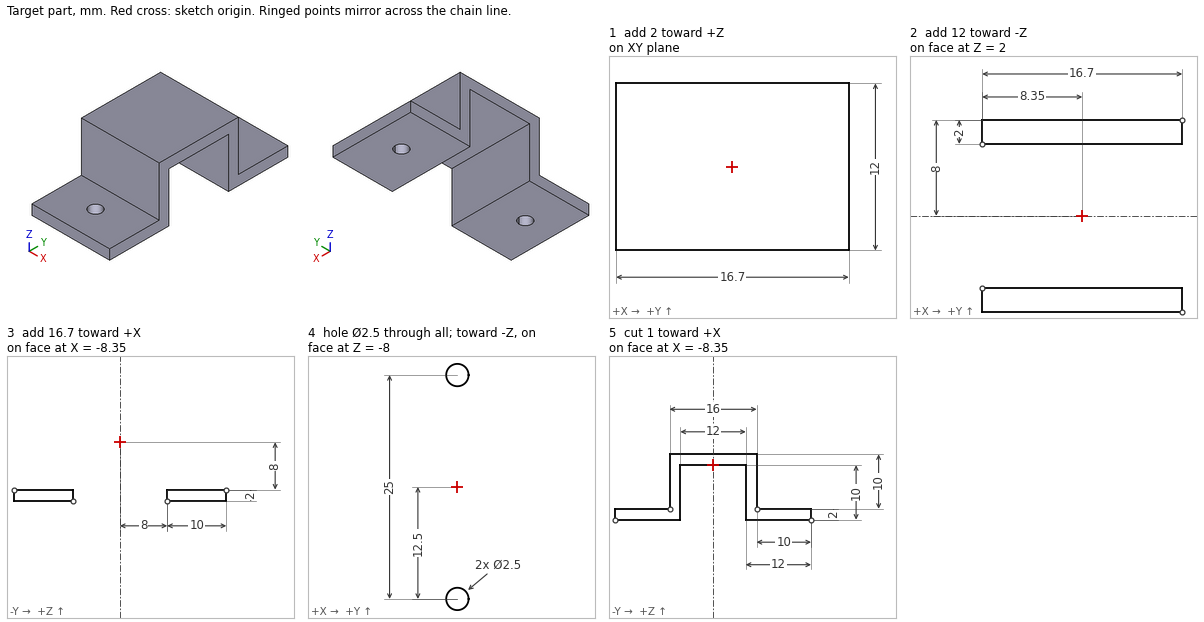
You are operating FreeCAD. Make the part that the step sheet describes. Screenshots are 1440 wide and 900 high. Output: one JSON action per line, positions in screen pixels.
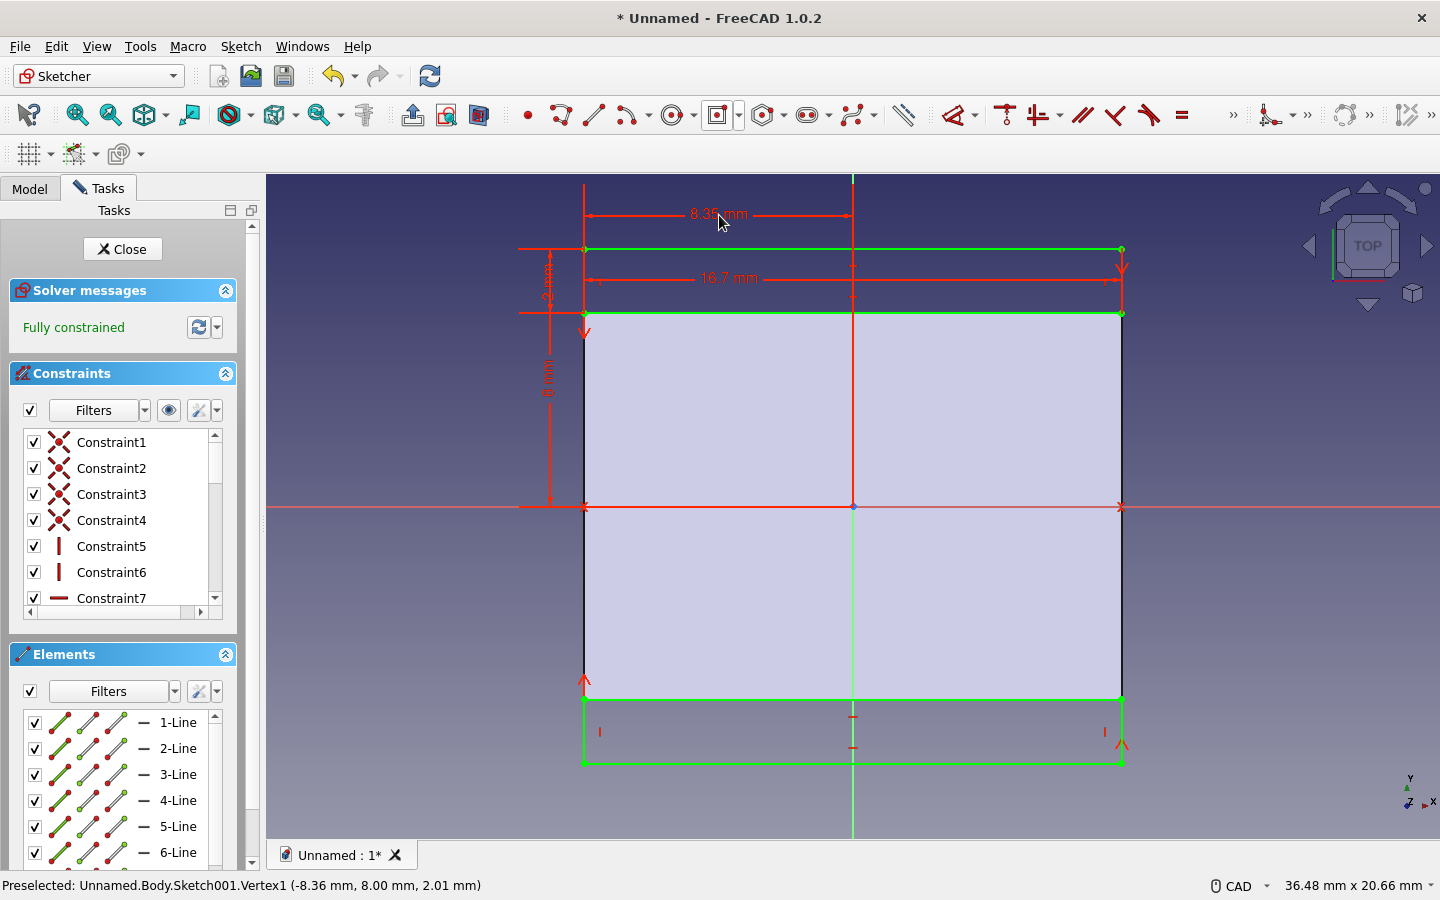
{"action": "left_click", "coordinate": [123, 249]}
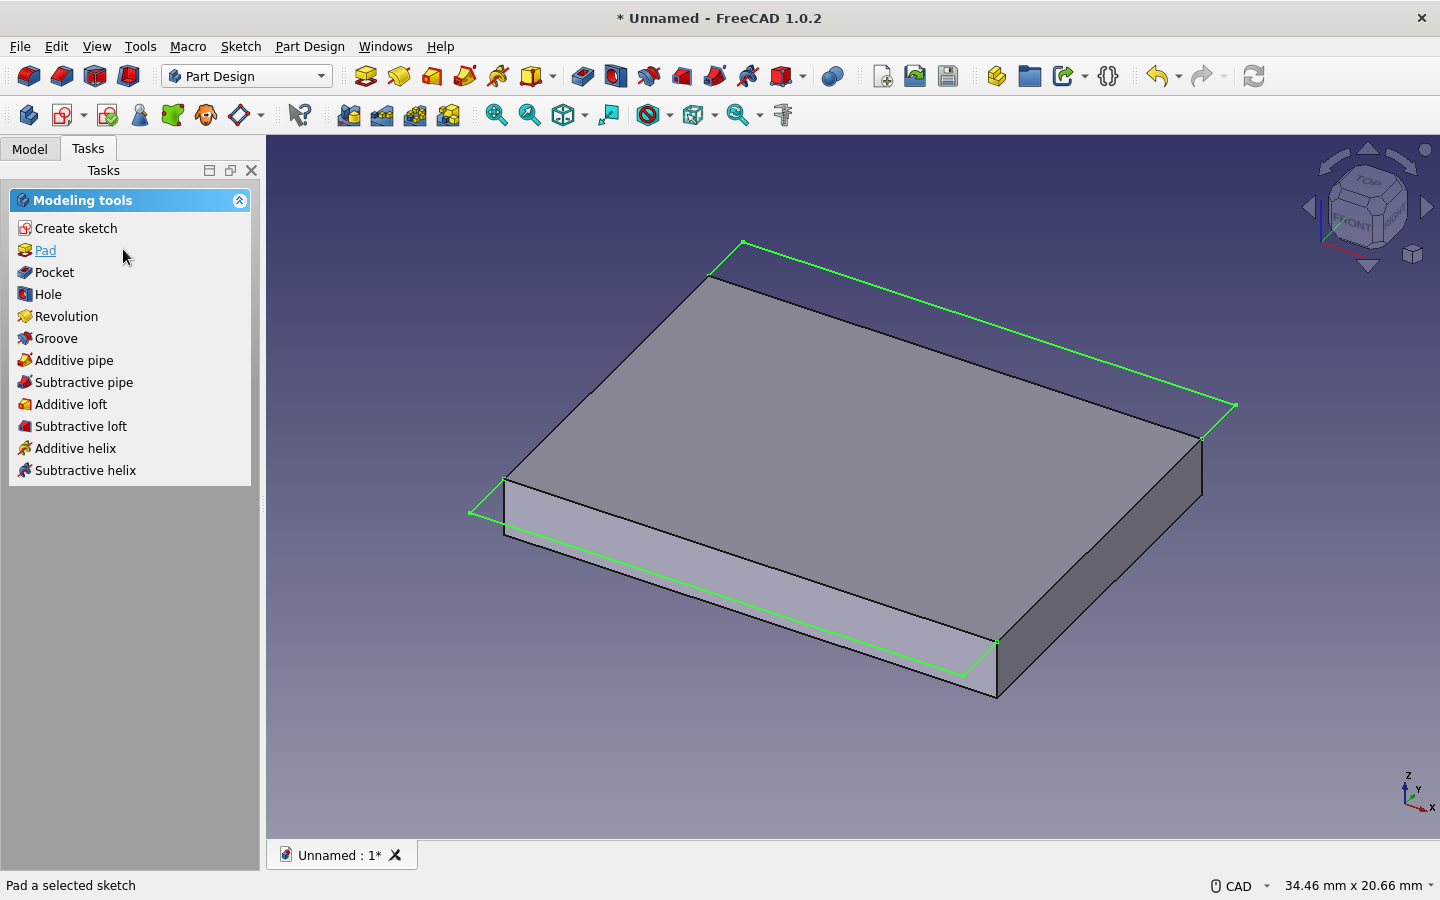
{"action": "left_click", "coordinate": [366, 76]}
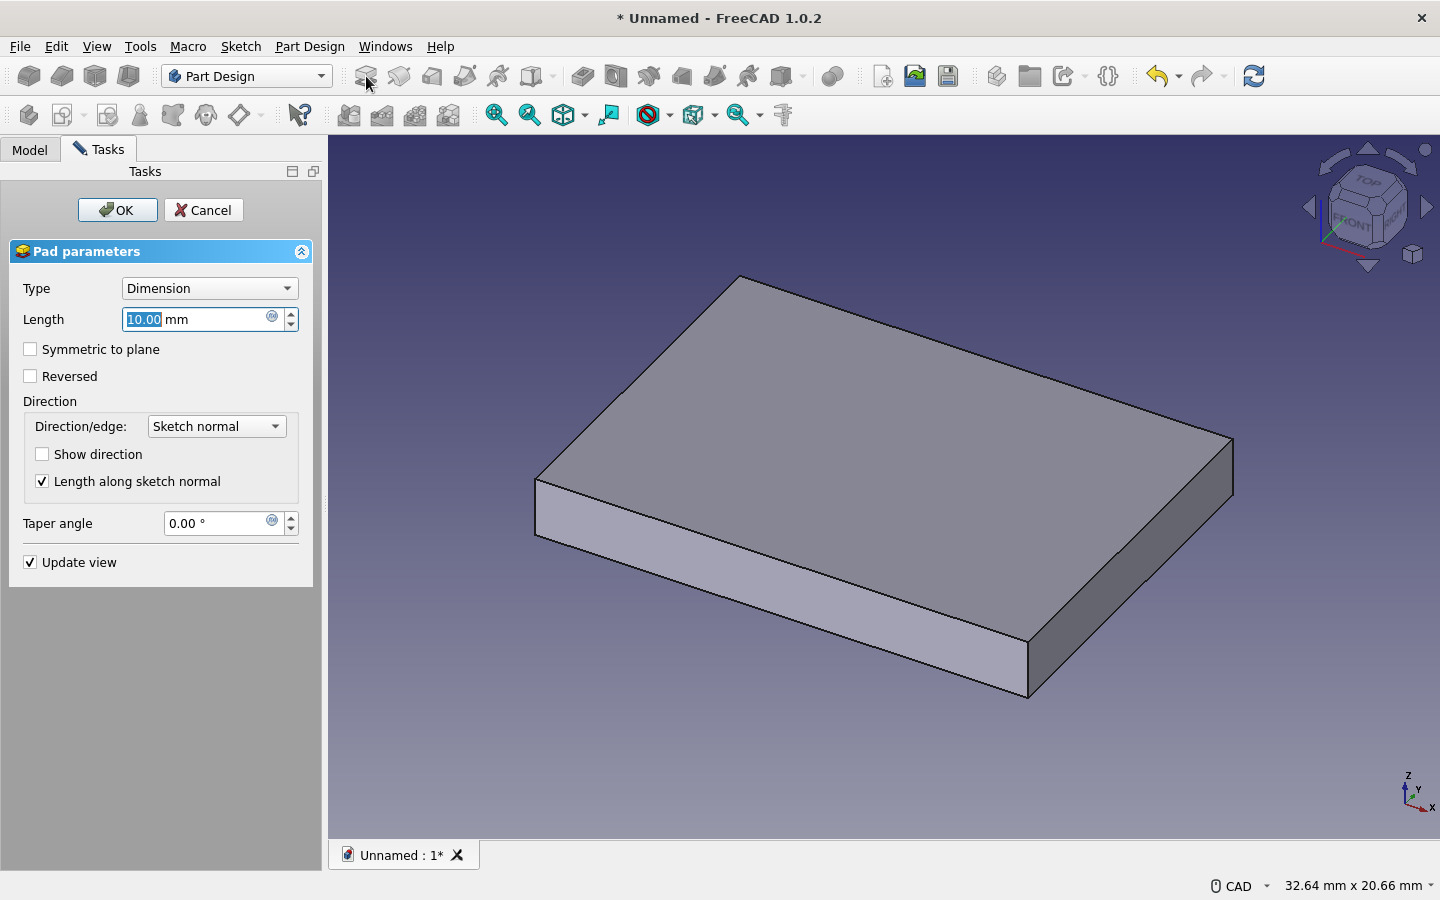
{"action": "type", "text": "12"}
{"action": "key", "text": "Tab"}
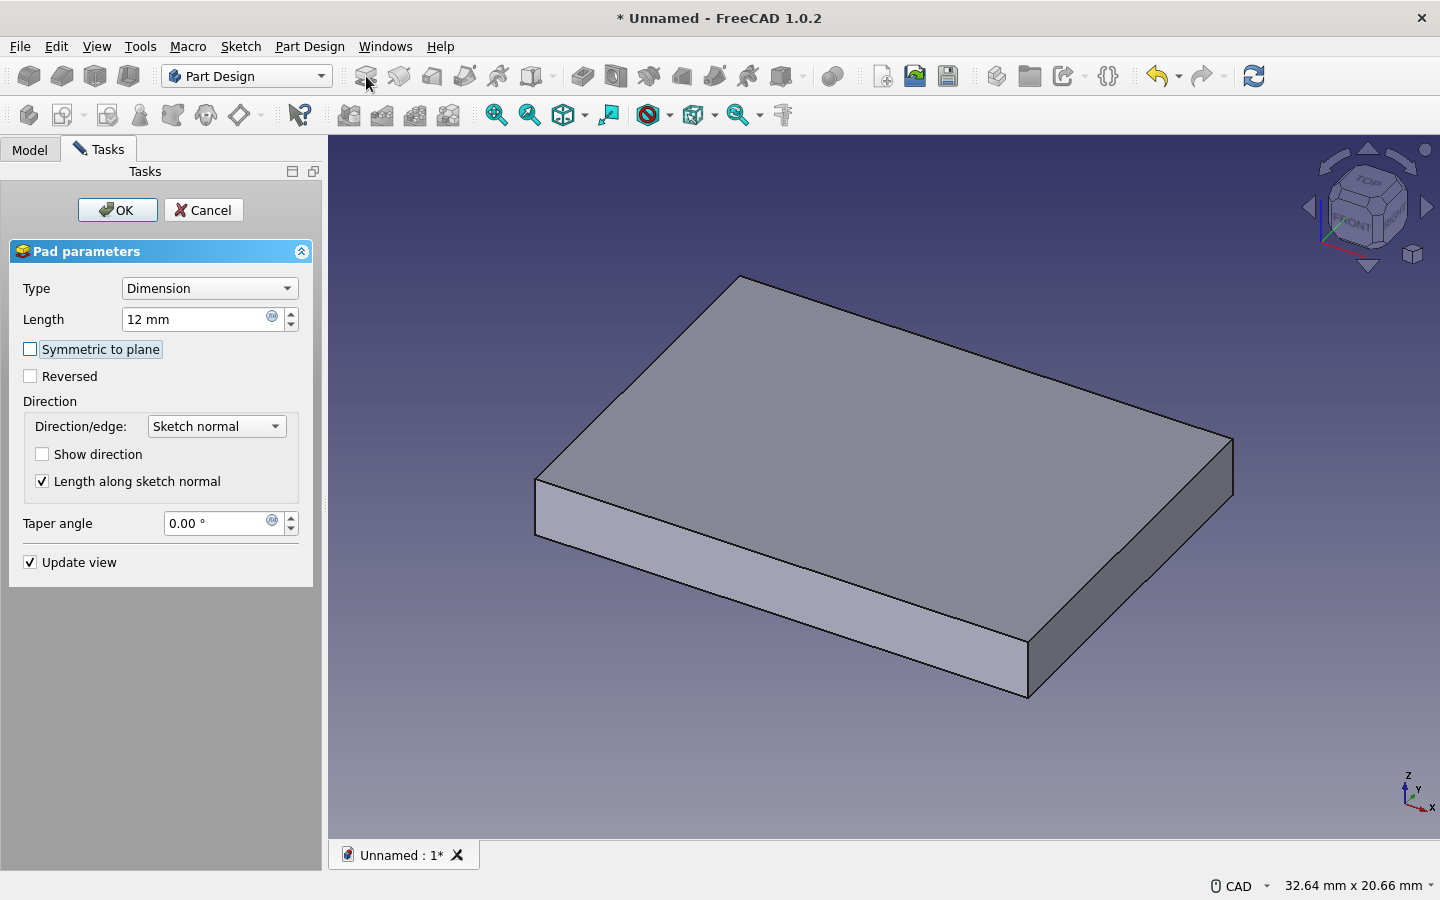
{"action": "left_click", "coordinate": [31, 376]}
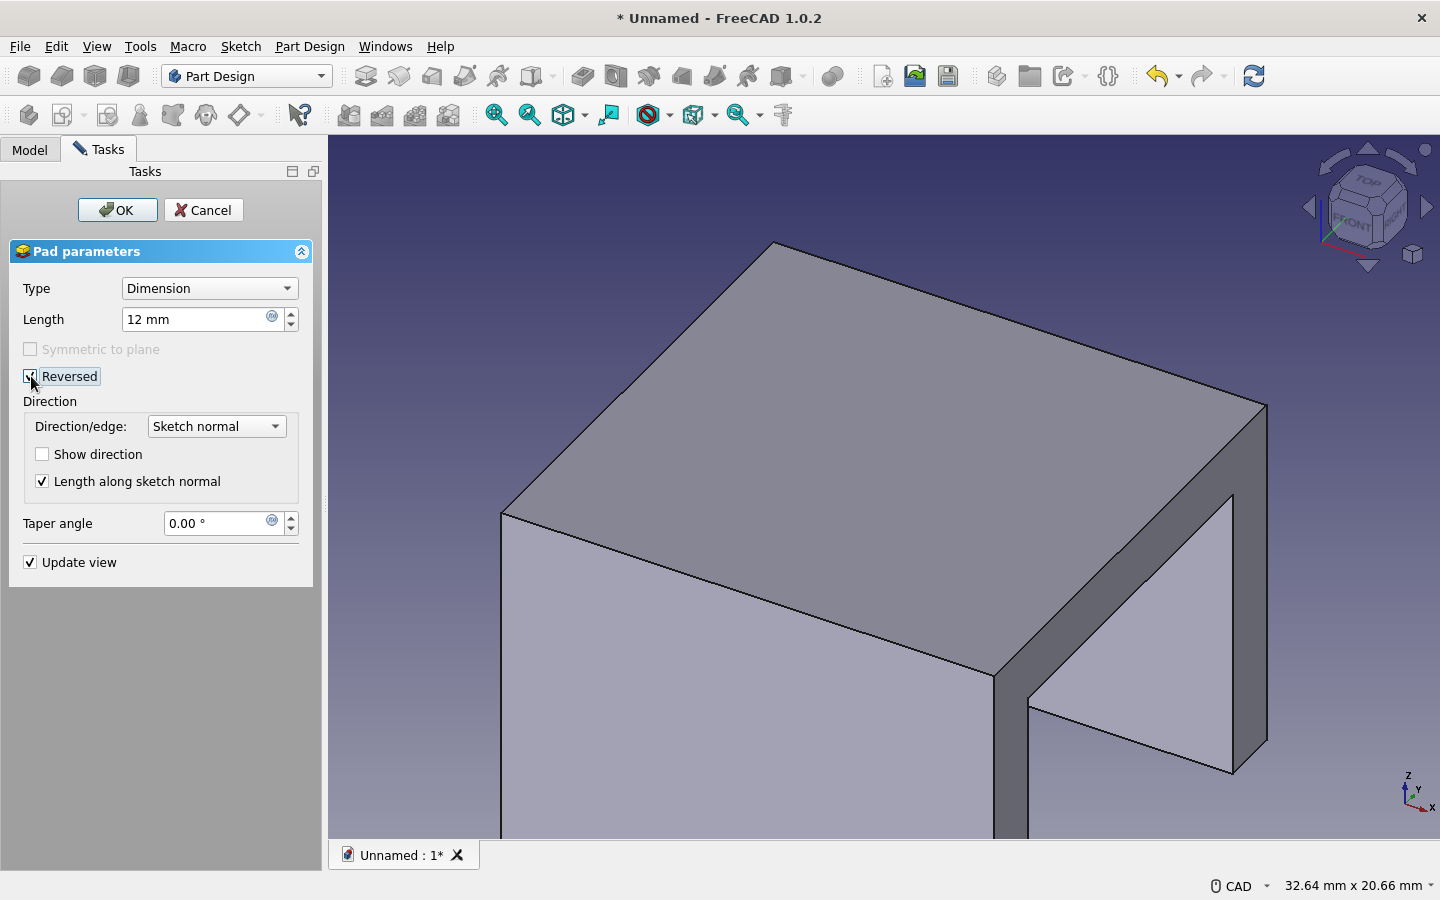
{"action": "left_click", "coordinate": [118, 210]}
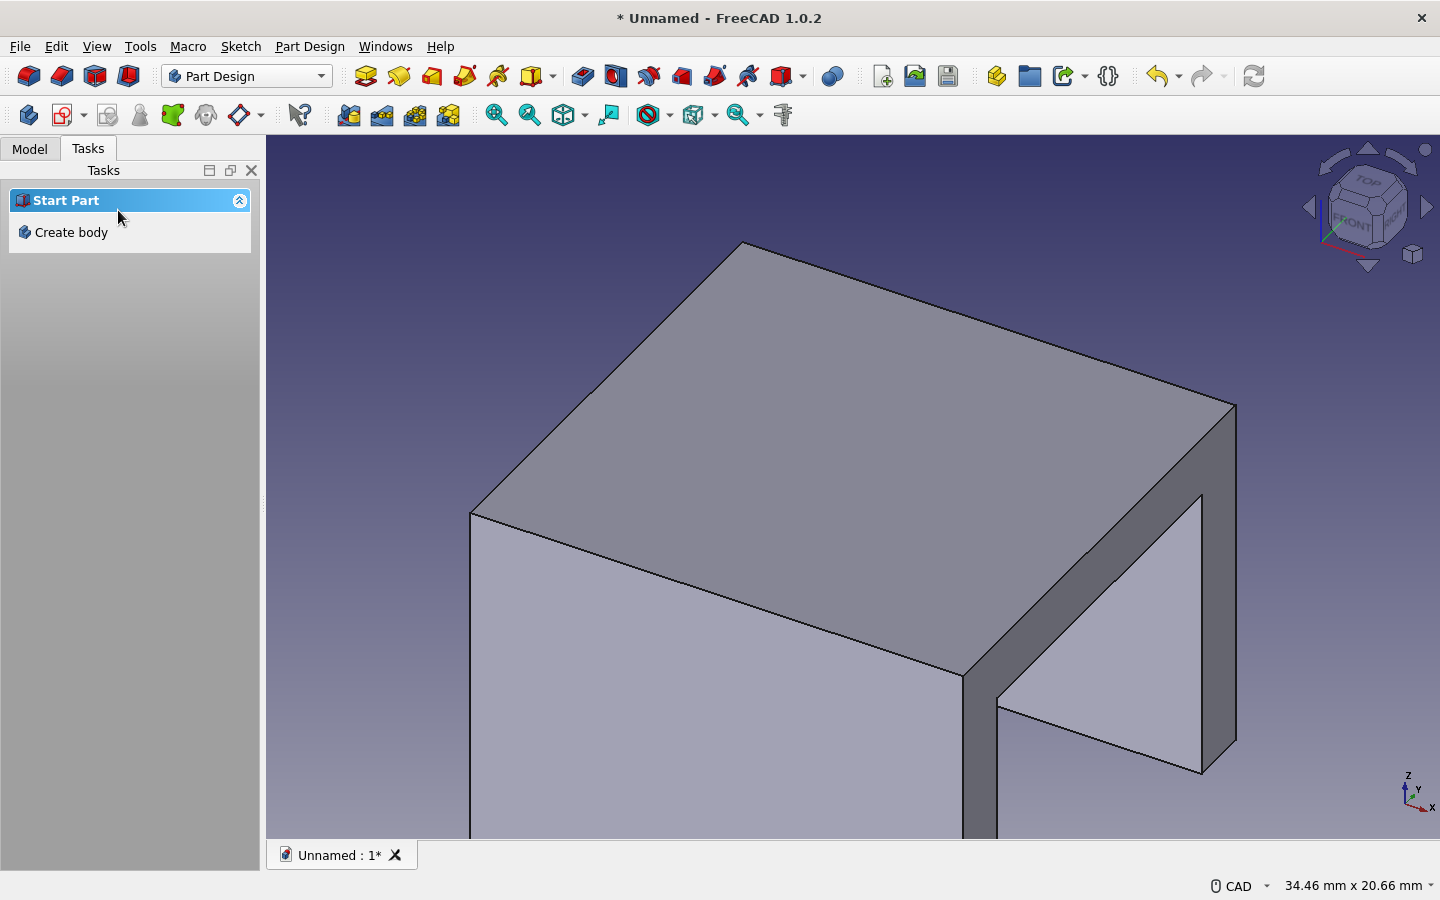
{"action": "left_click", "coordinate": [497, 116]}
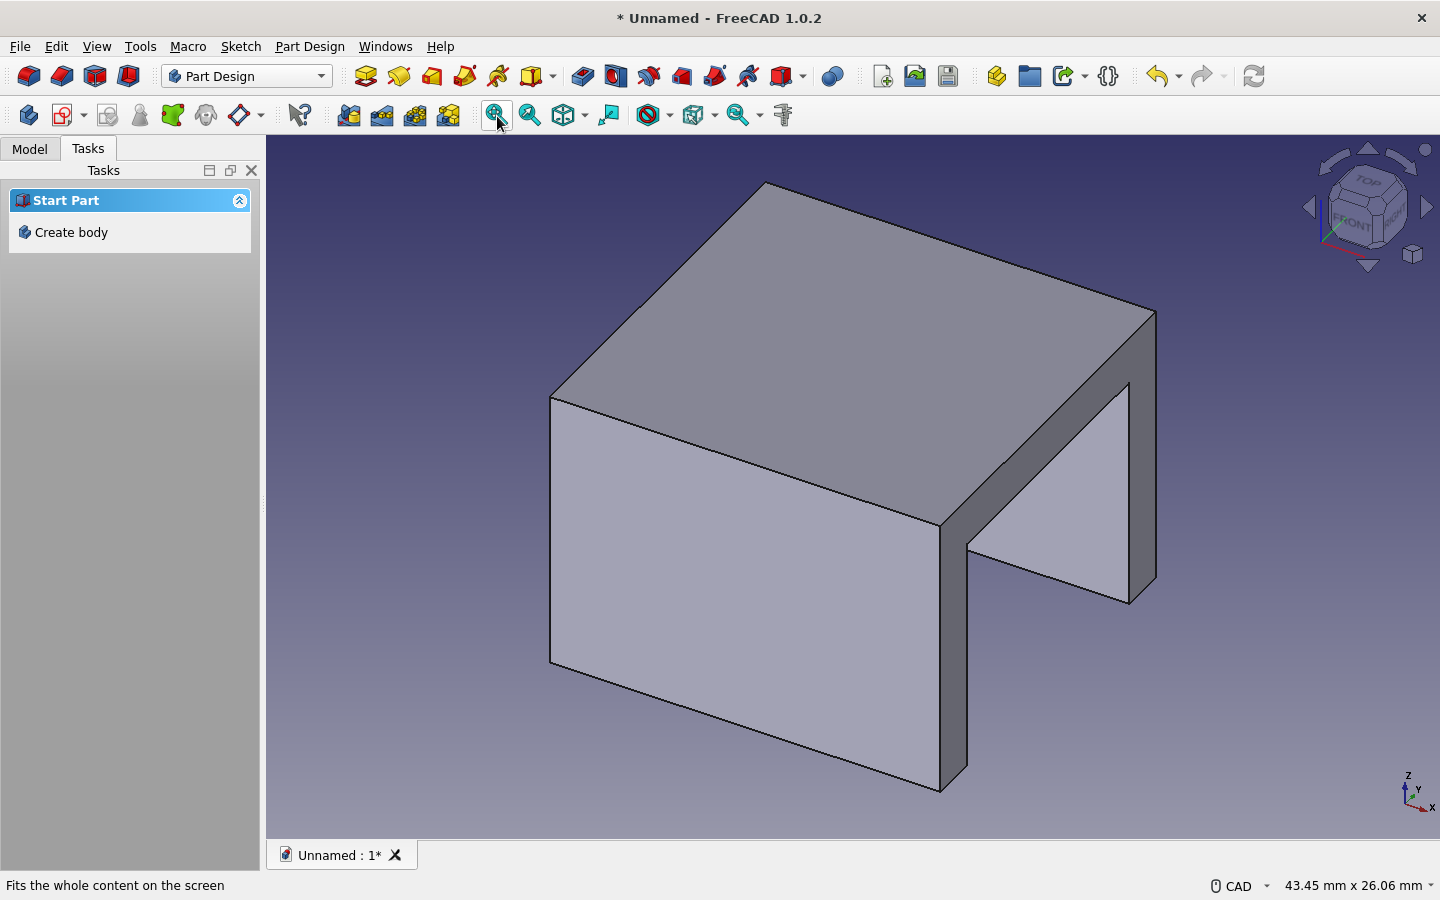
{"action": "key", "text": "6"}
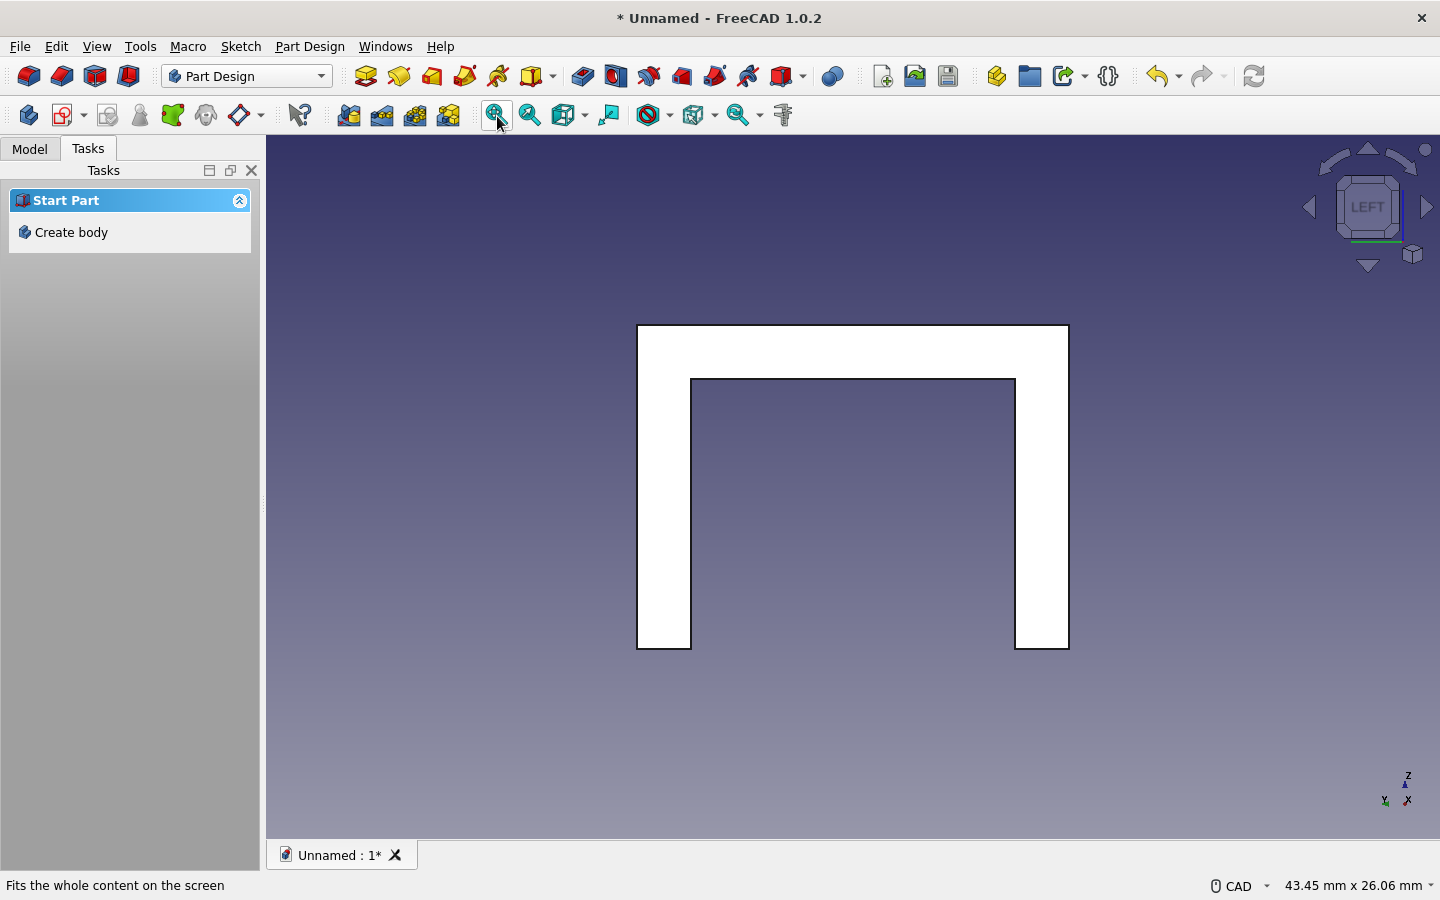
{"action": "left_click", "coordinate": [668, 393]}